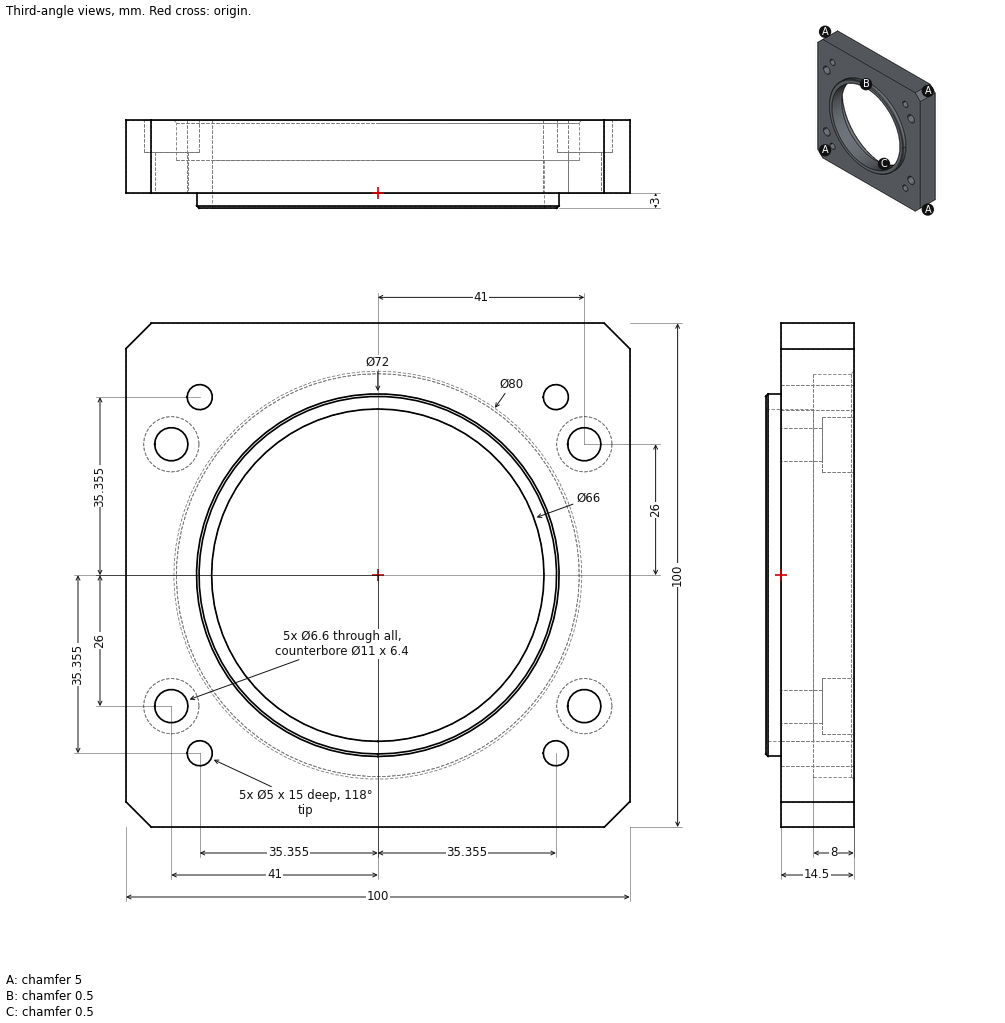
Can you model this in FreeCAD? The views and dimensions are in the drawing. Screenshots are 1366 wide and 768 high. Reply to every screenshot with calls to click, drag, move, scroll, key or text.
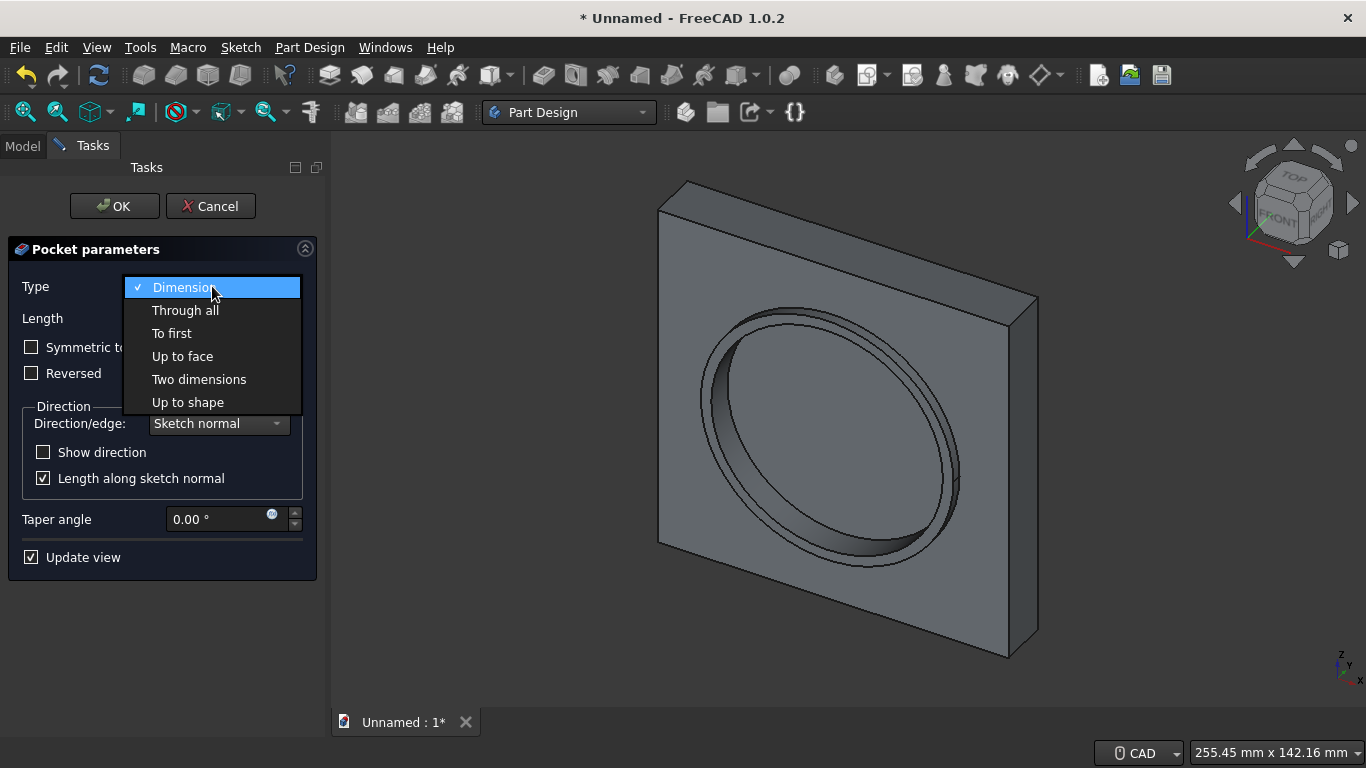
click(212, 310)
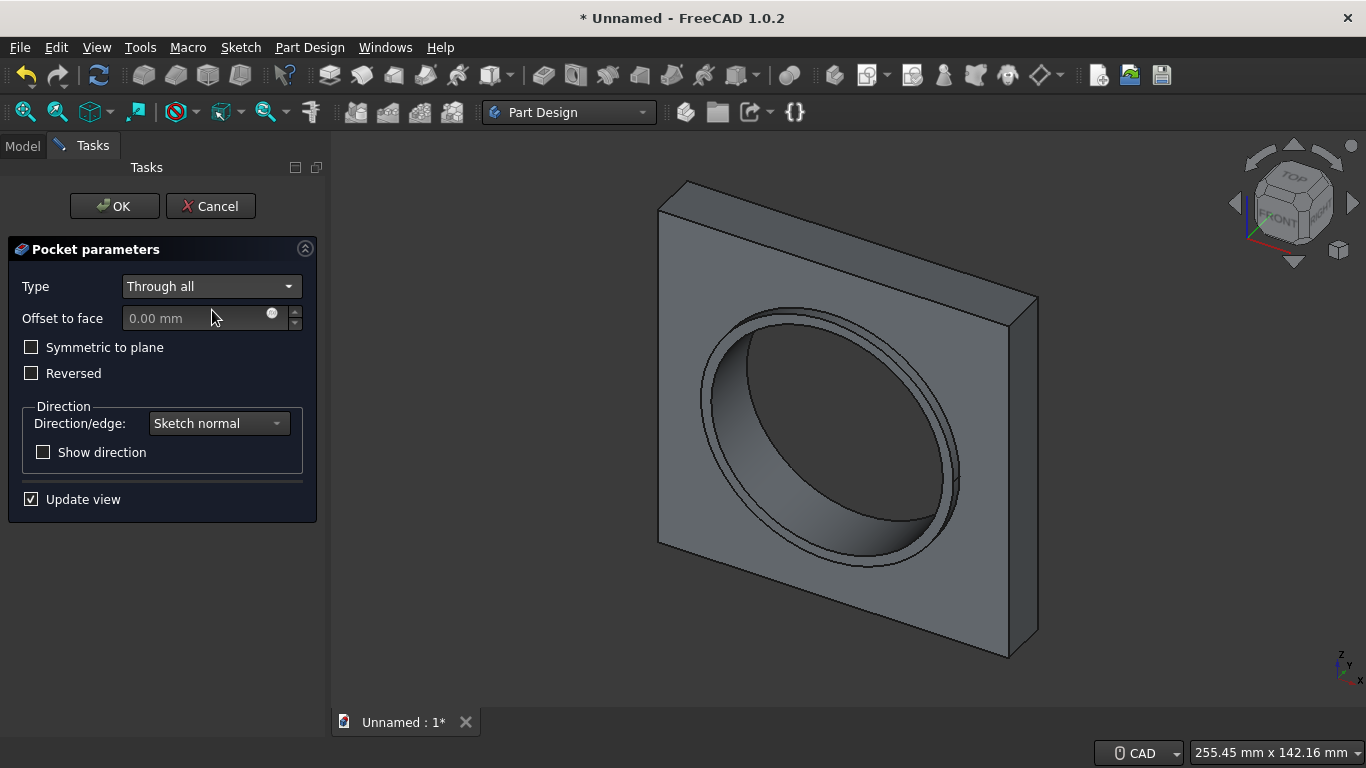
click(115, 206)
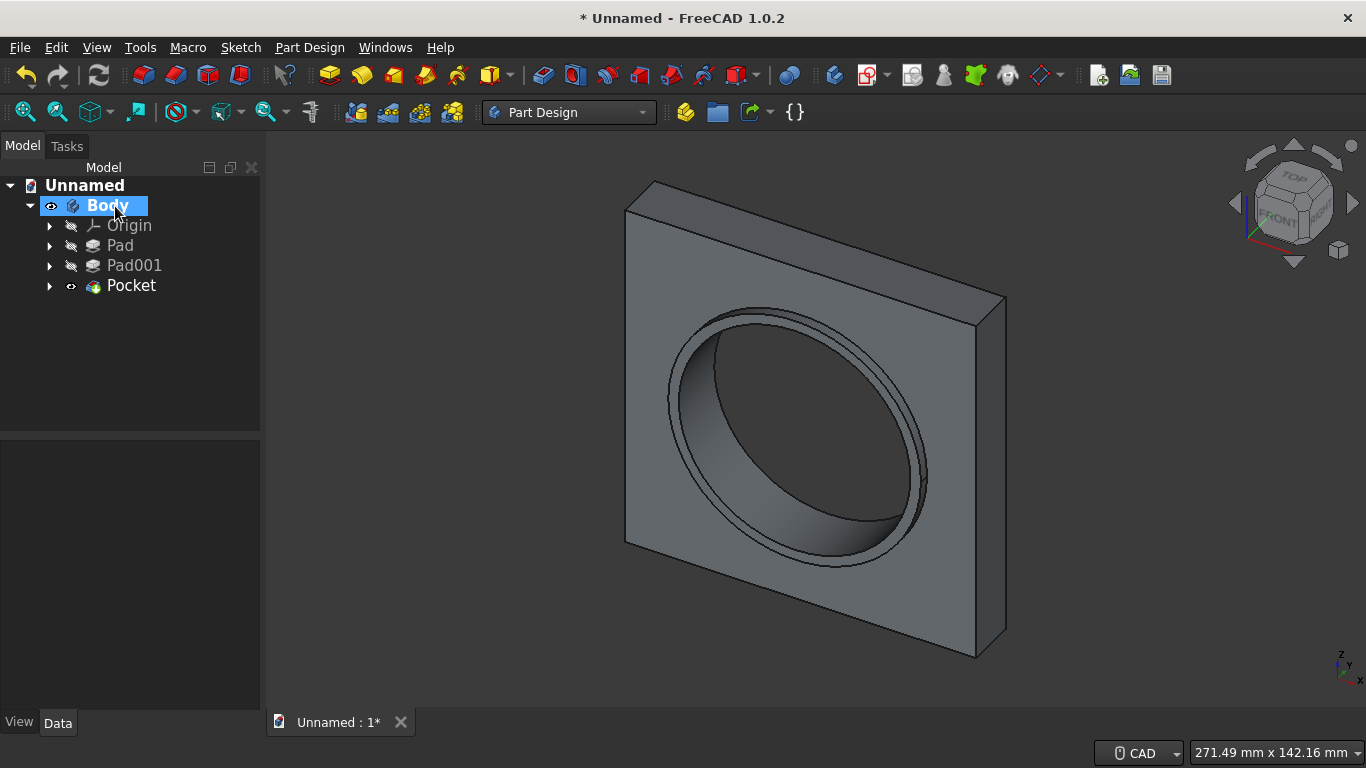
click(991, 311)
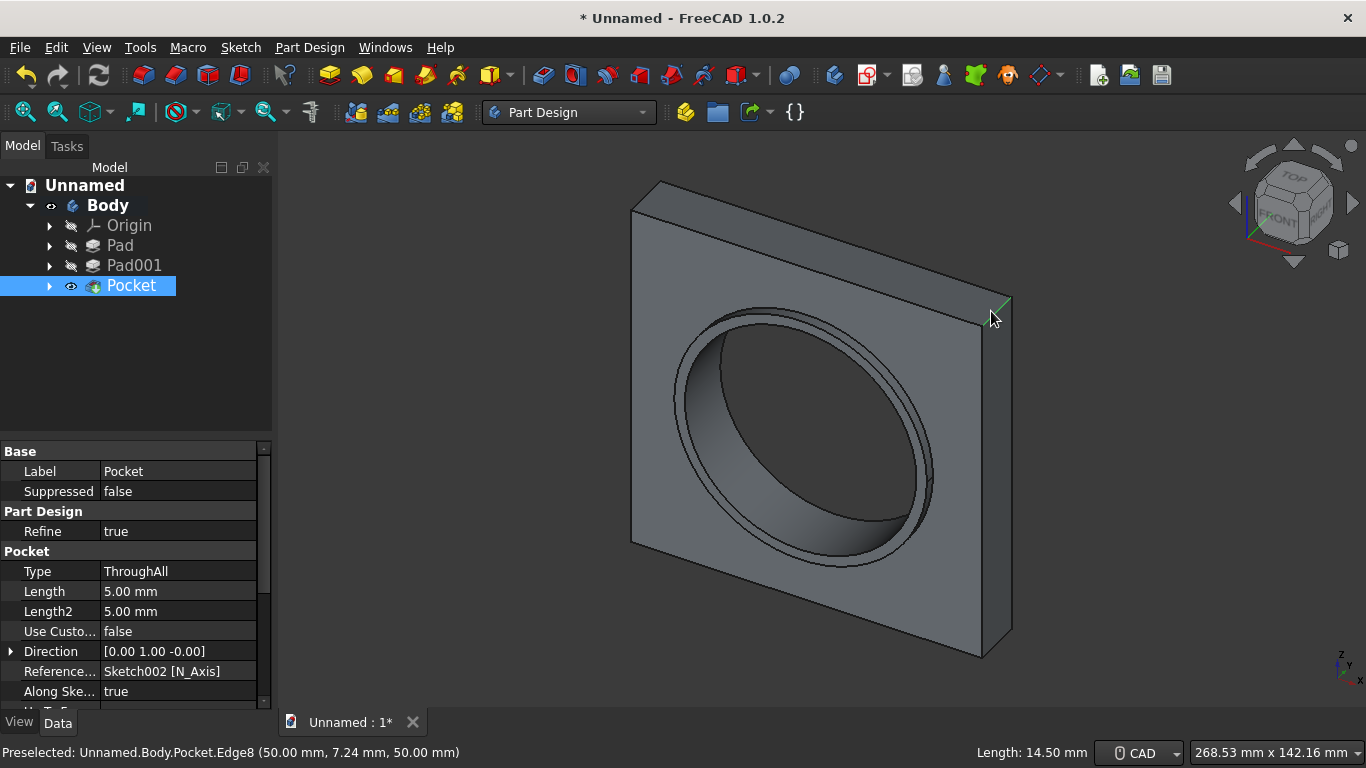
key(0)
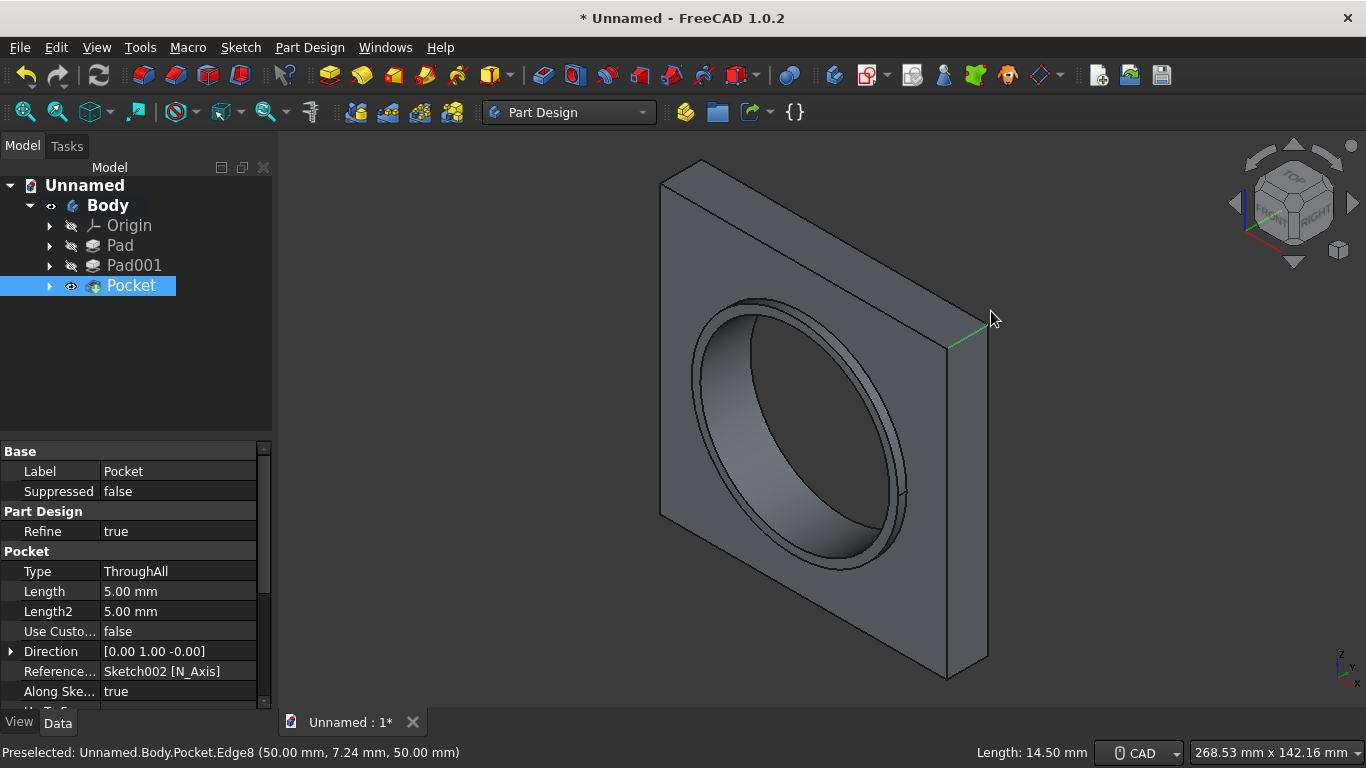
key(2)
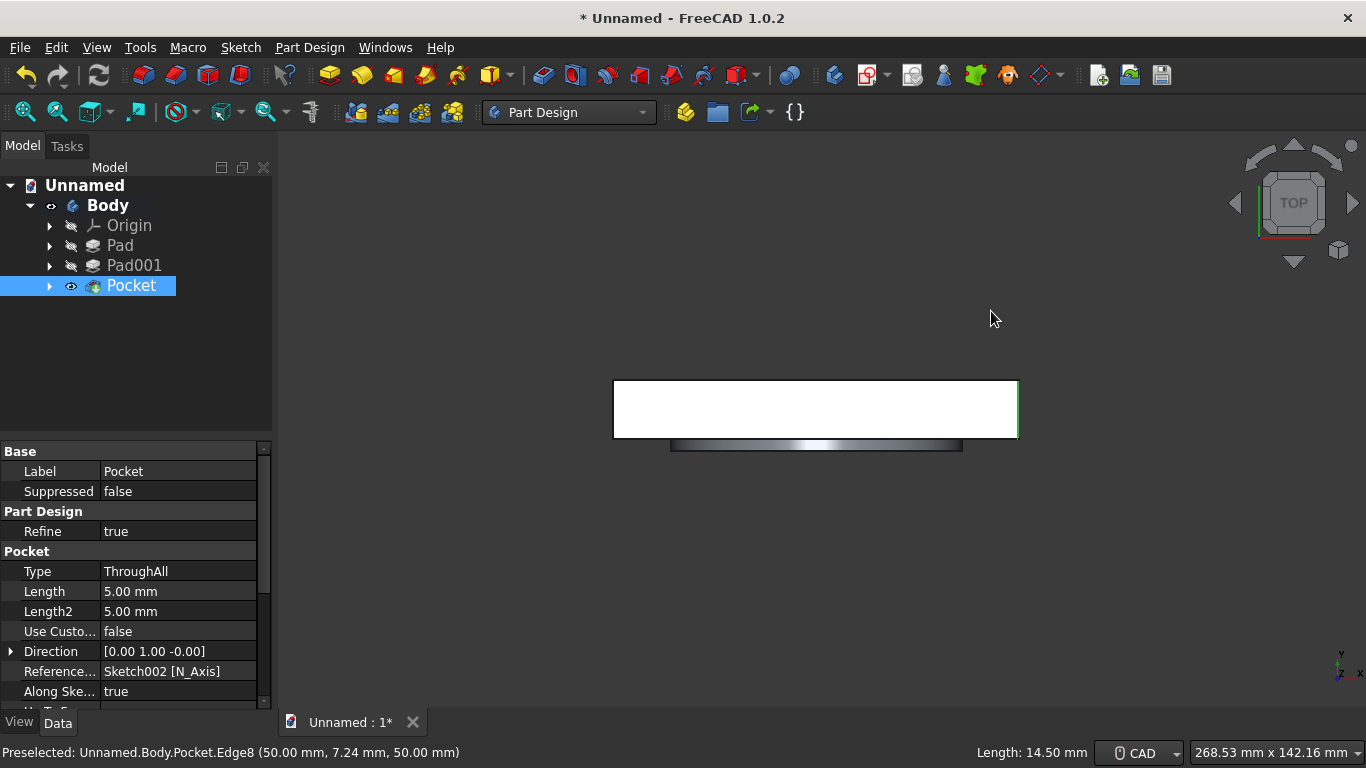
key(v)
key(f)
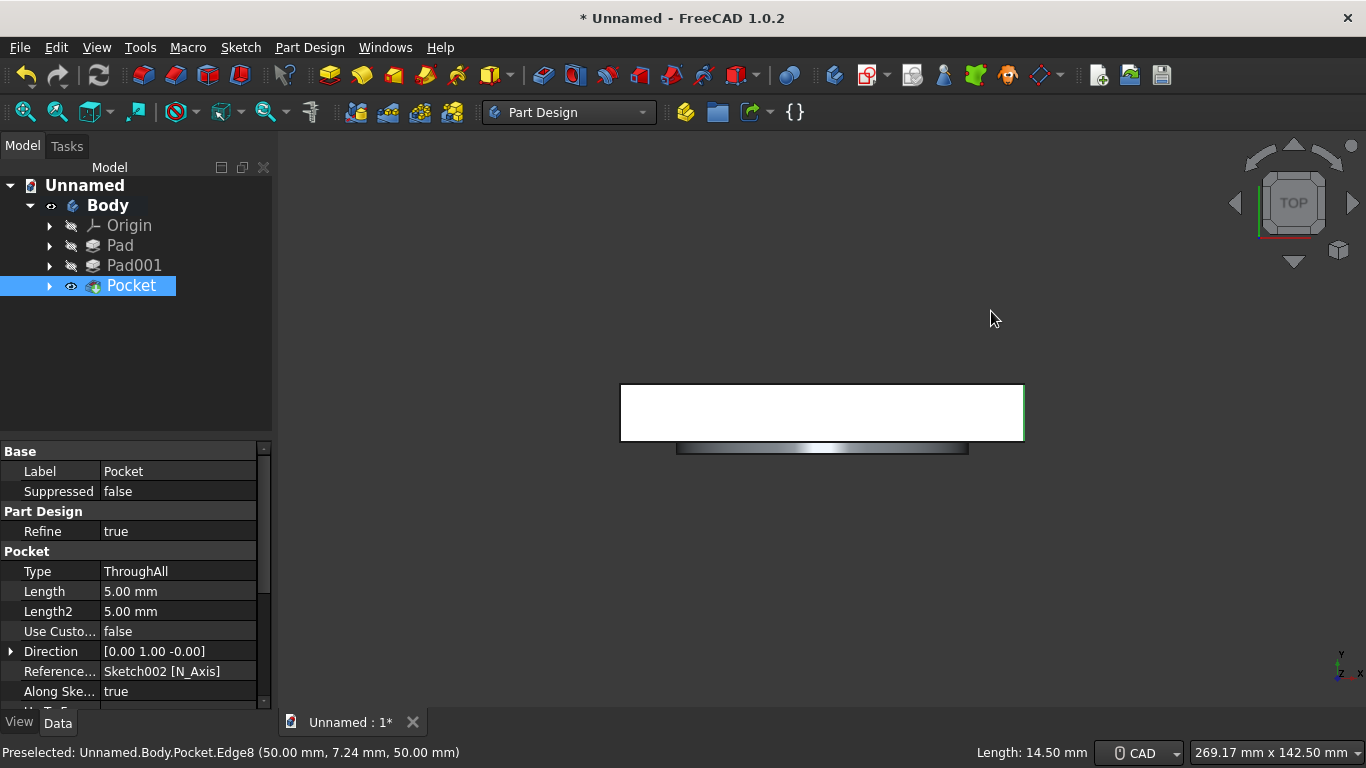
click(620, 412, ctrl)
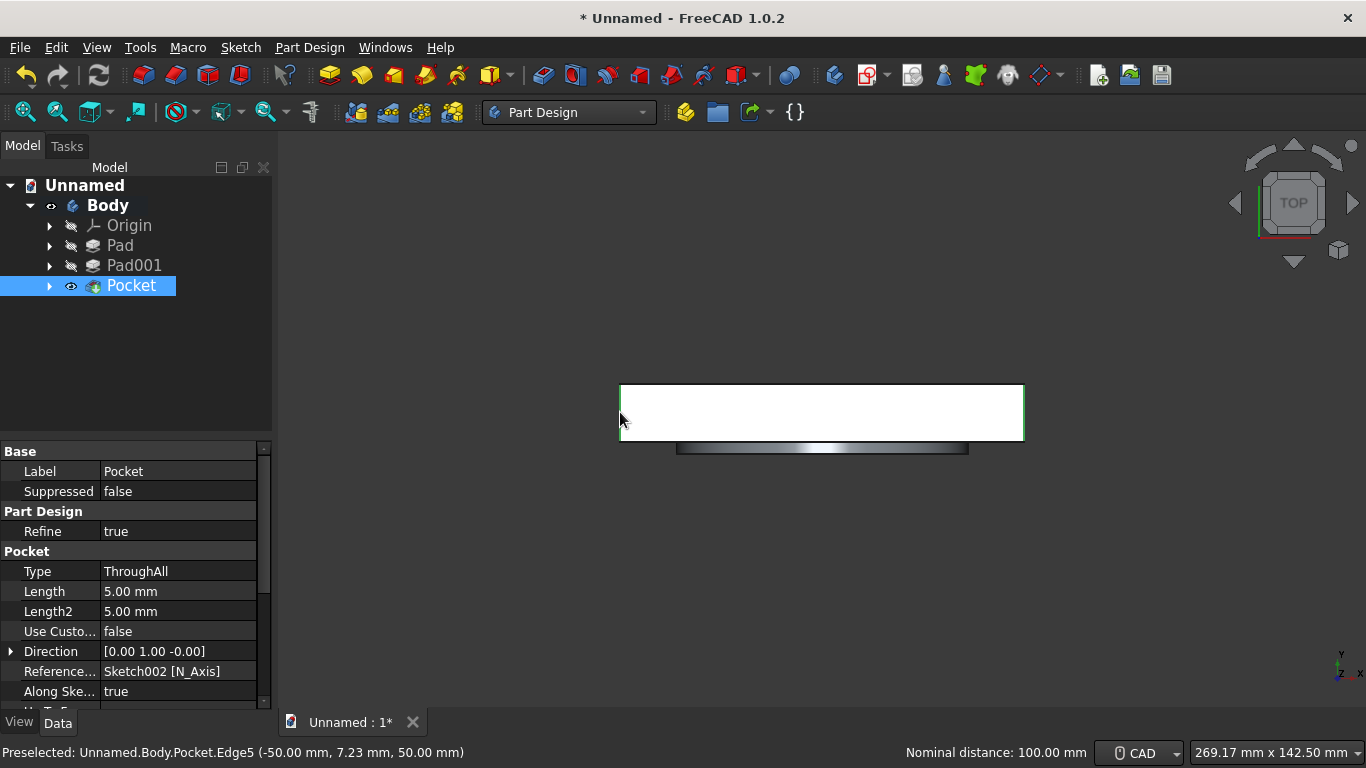
key(1)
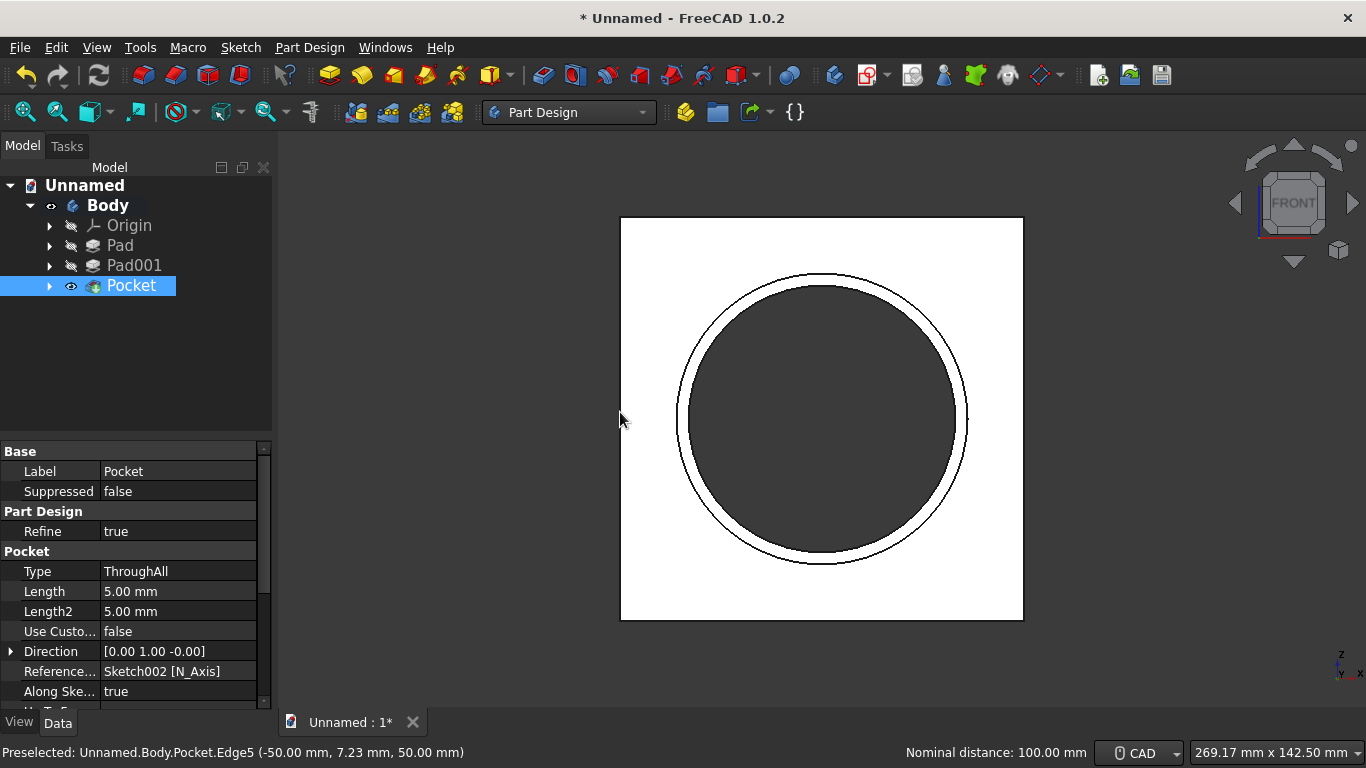
key(3)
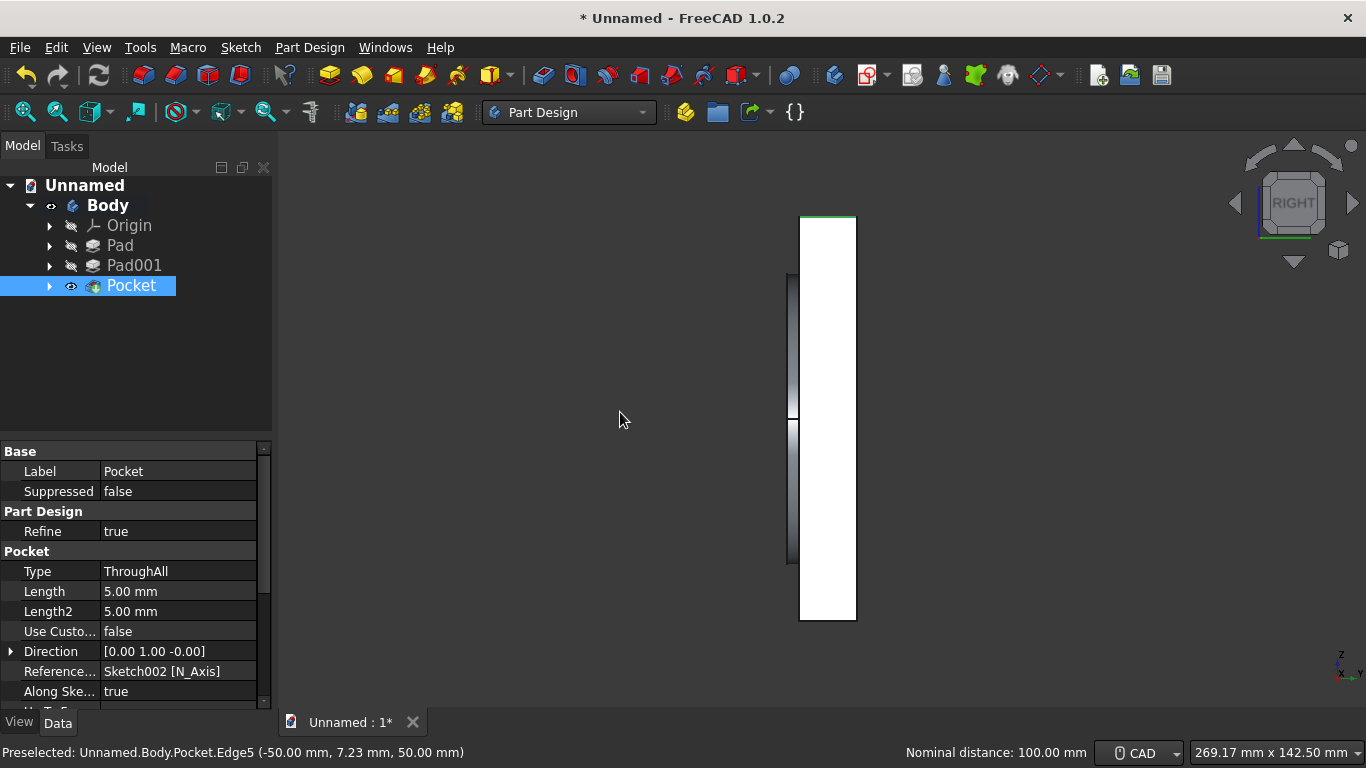
click(828, 620, ctrl)